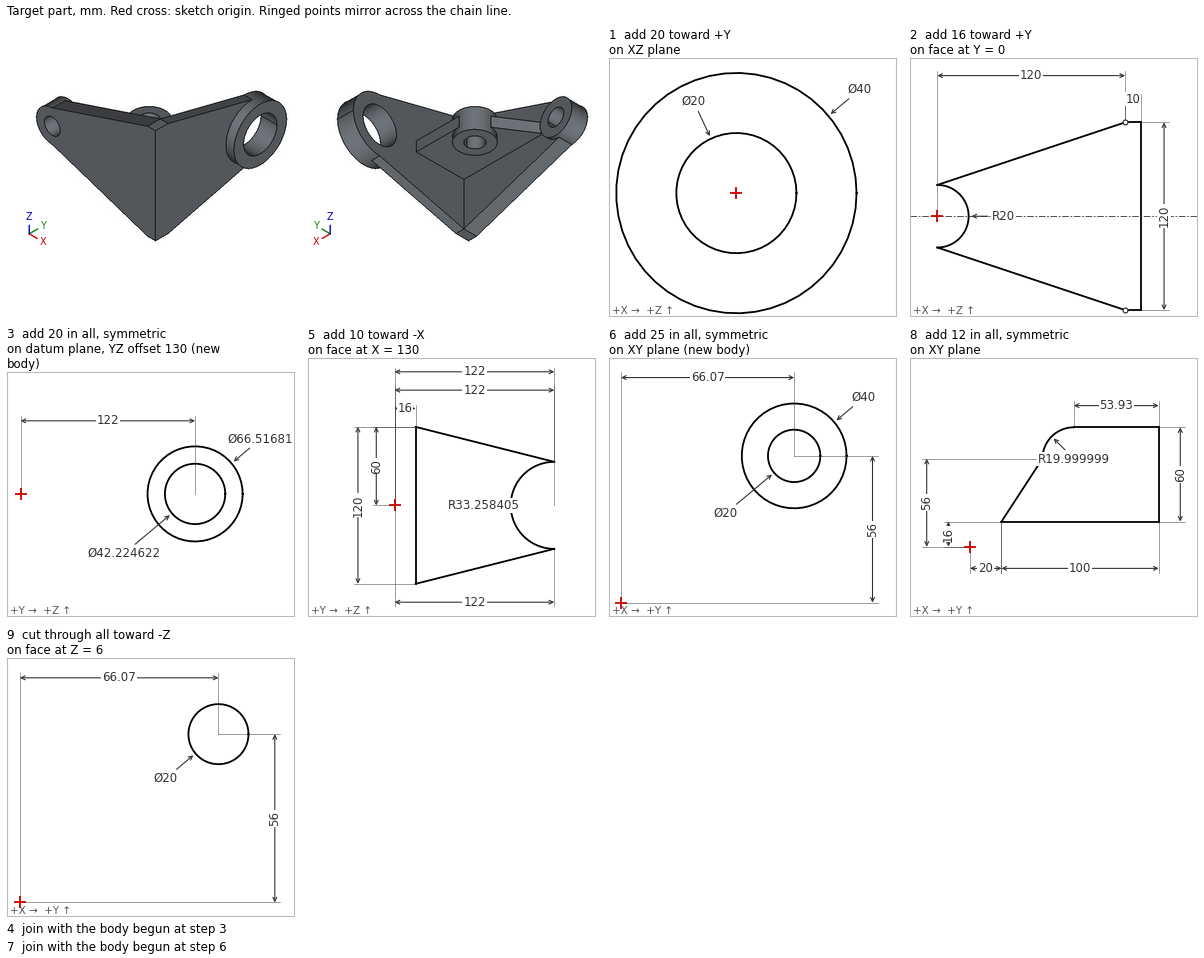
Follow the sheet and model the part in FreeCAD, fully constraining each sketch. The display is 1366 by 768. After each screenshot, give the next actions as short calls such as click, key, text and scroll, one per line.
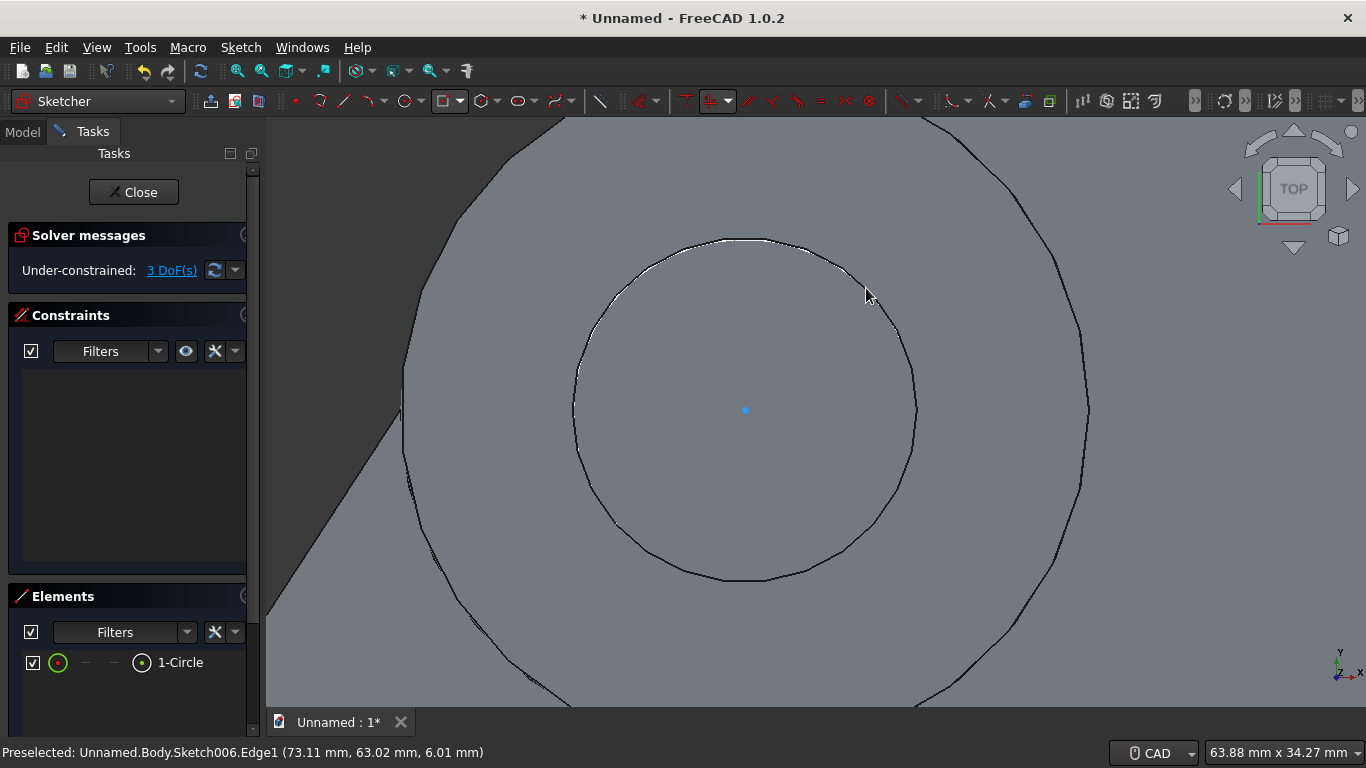
click(640, 102)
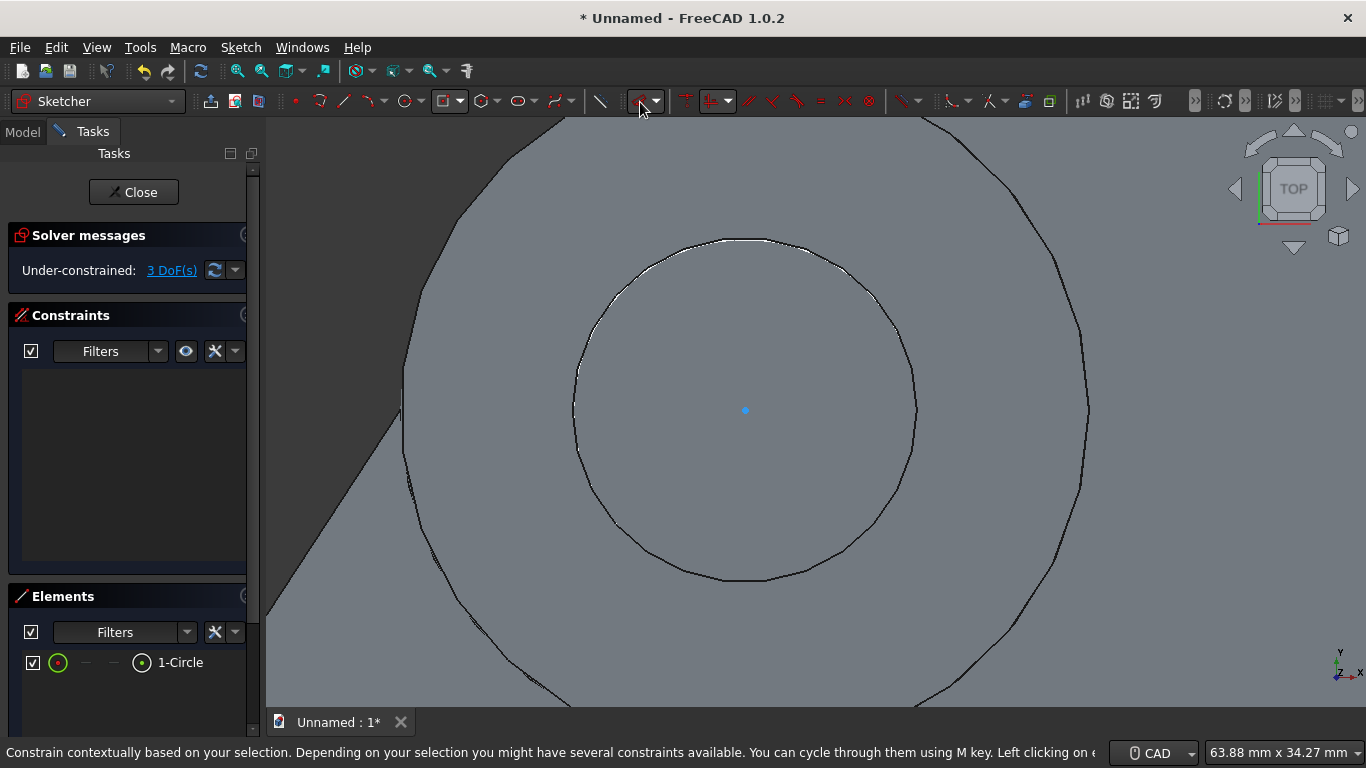
click(866, 289)
click(889, 266)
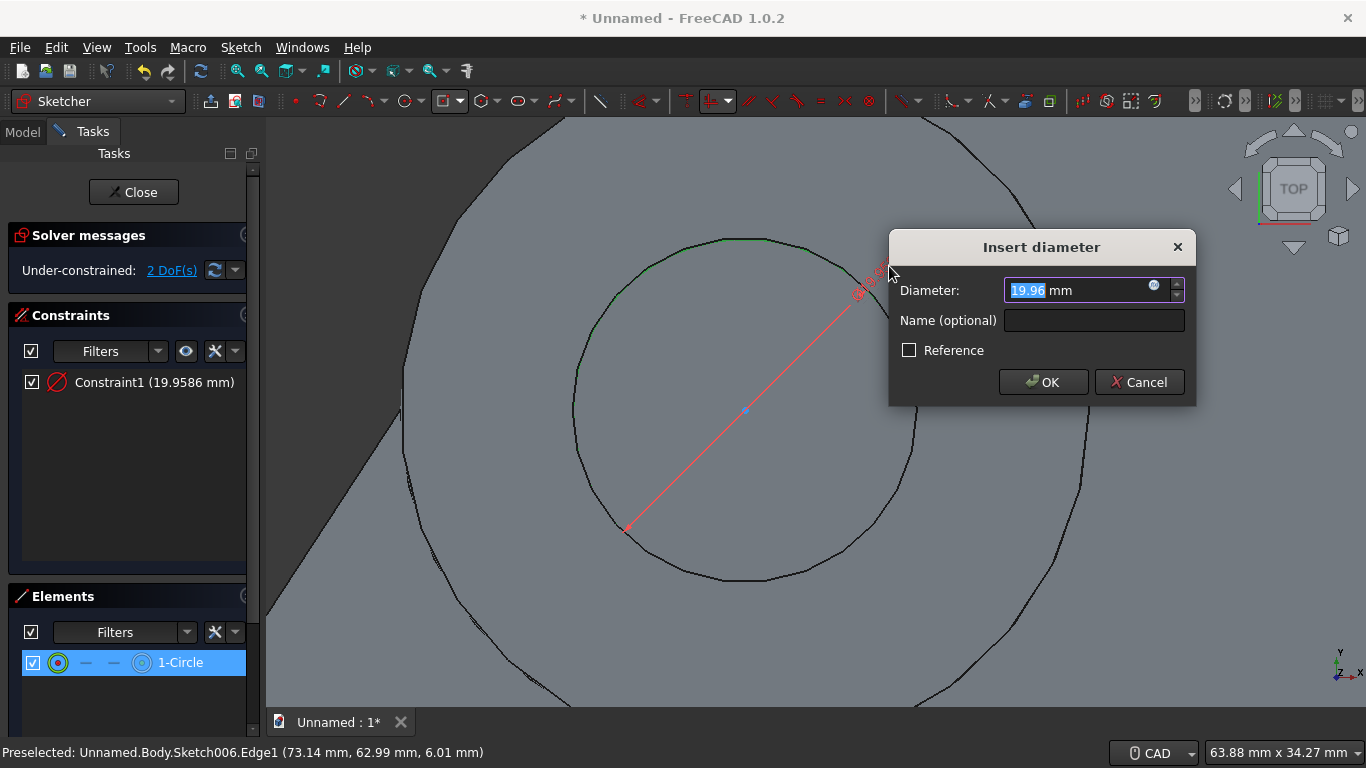
text(20)
key(Return)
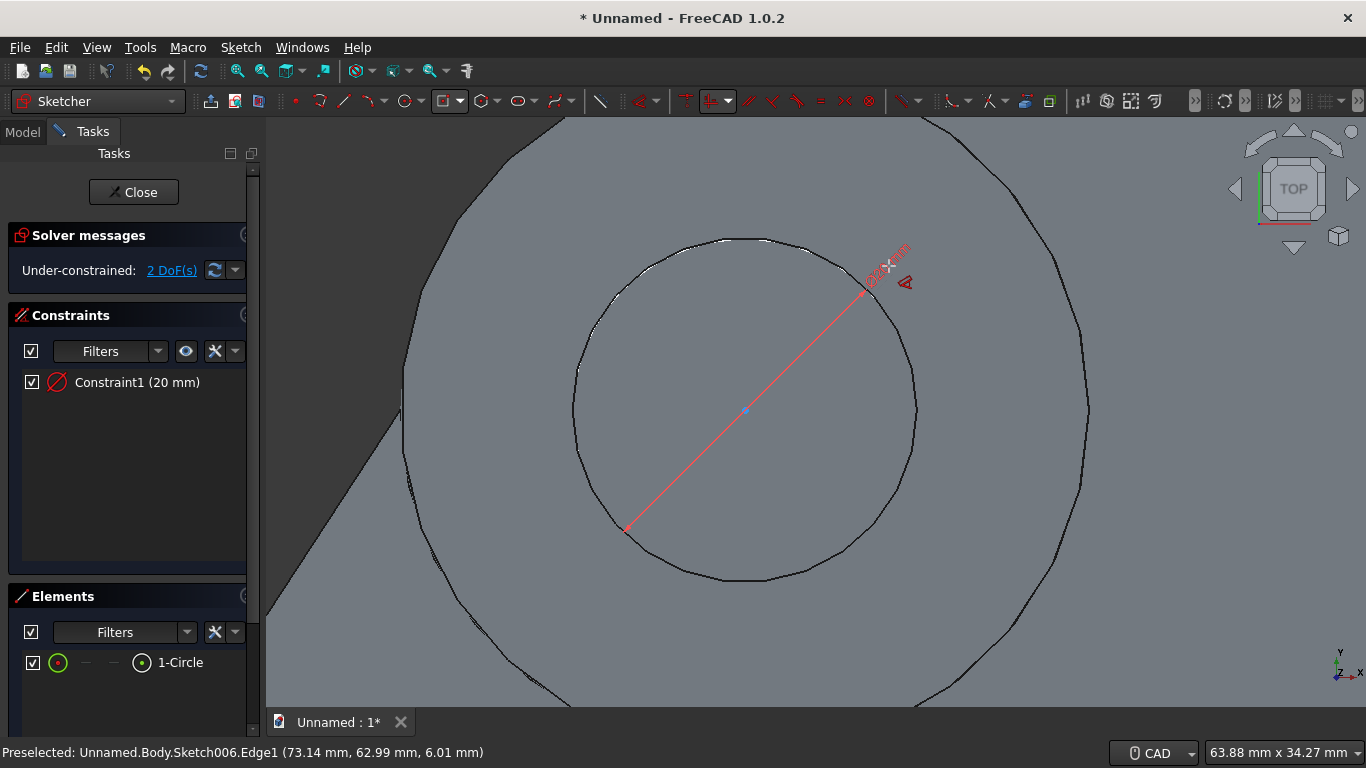
click(745, 411)
click(779, 545)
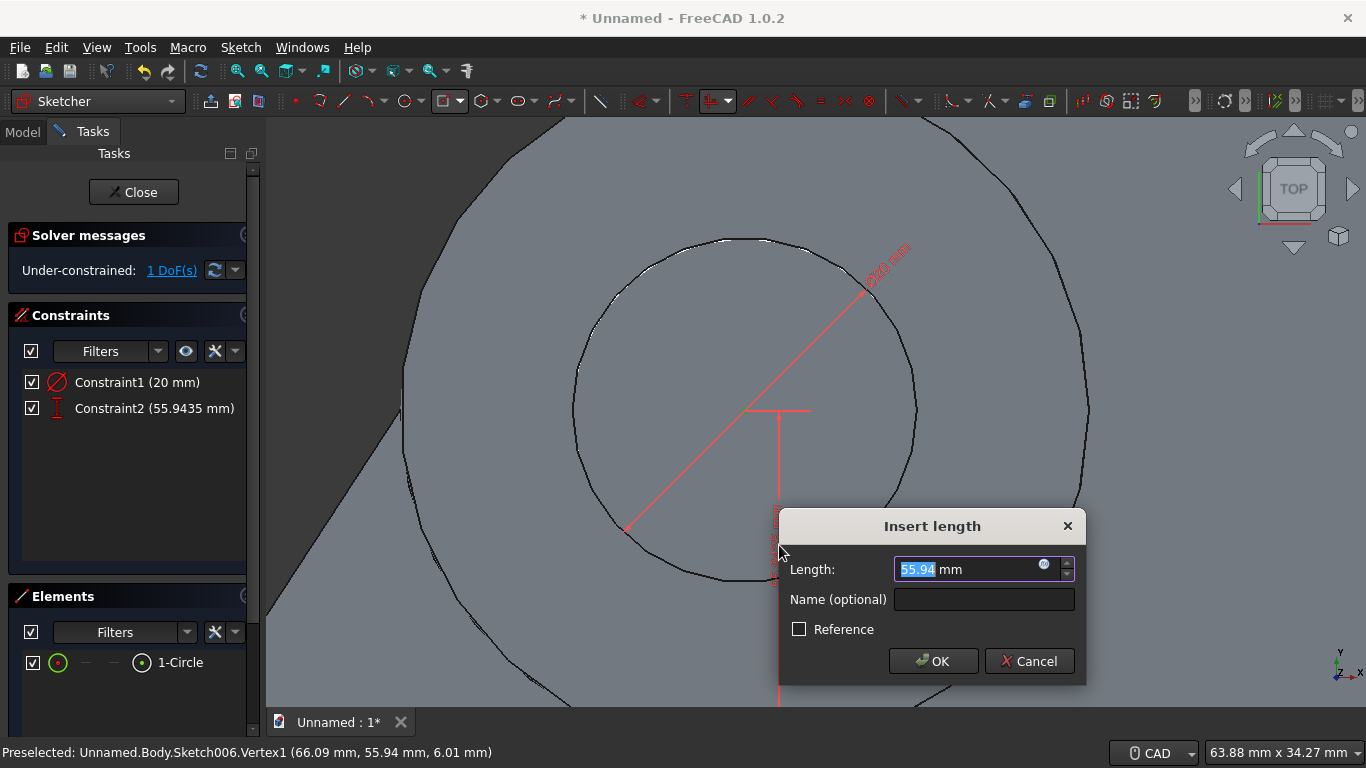
text(56)
key(Return)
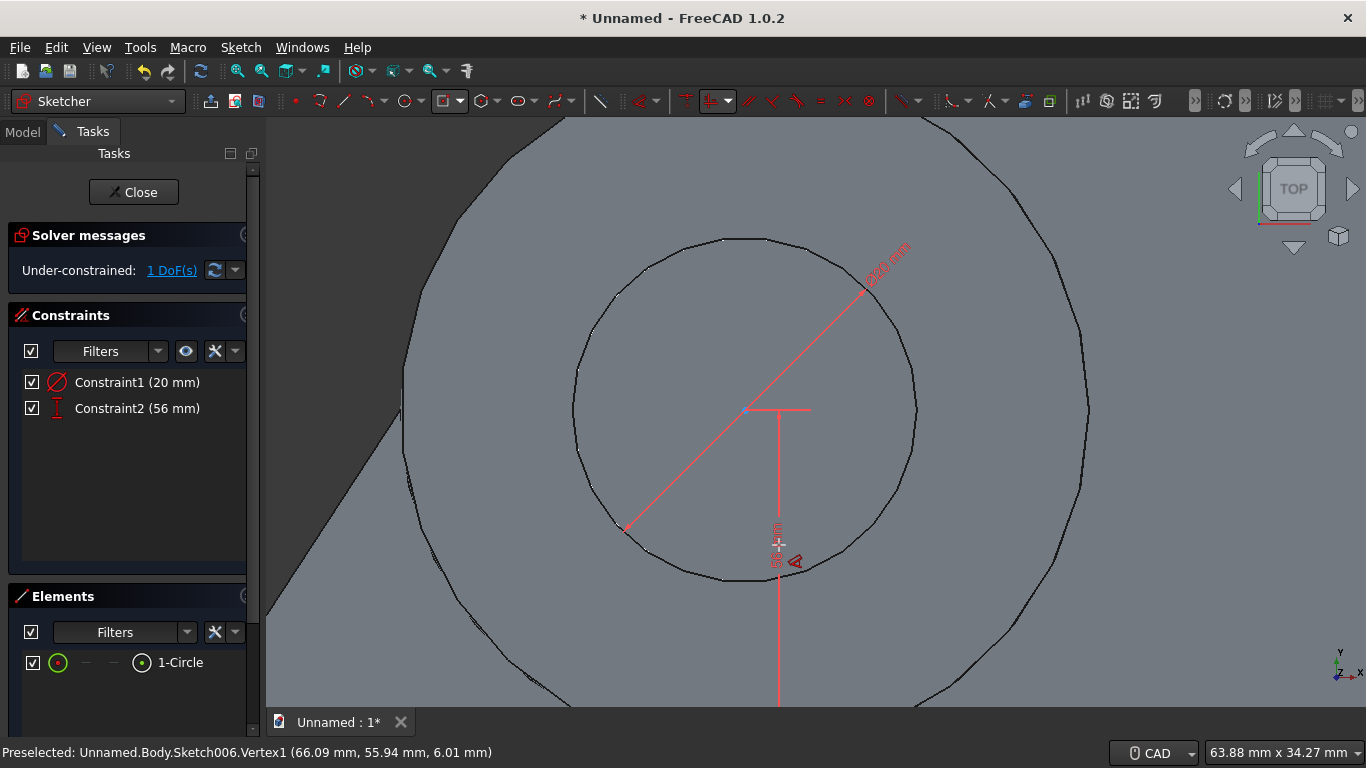
click(745, 410)
click(519, 376)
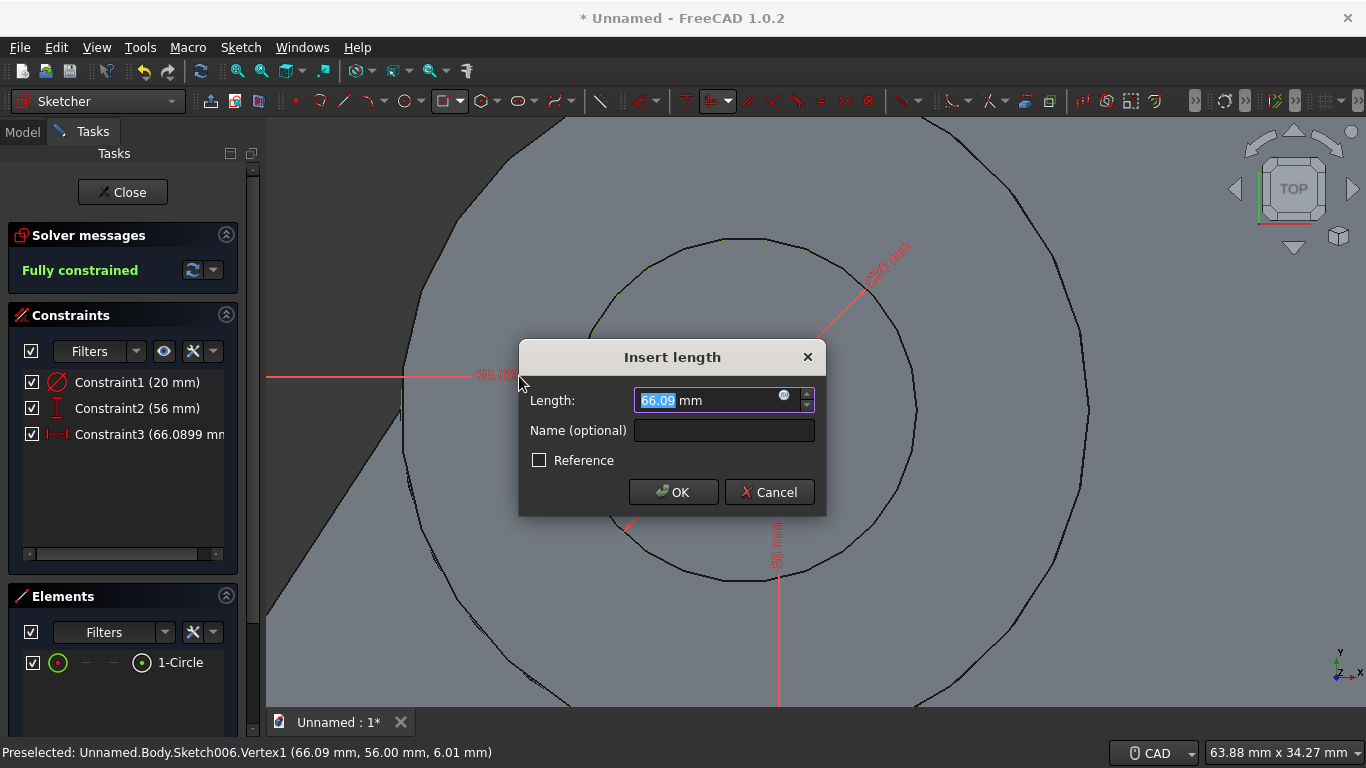
text(66.07)
key(Return)
key(Escape)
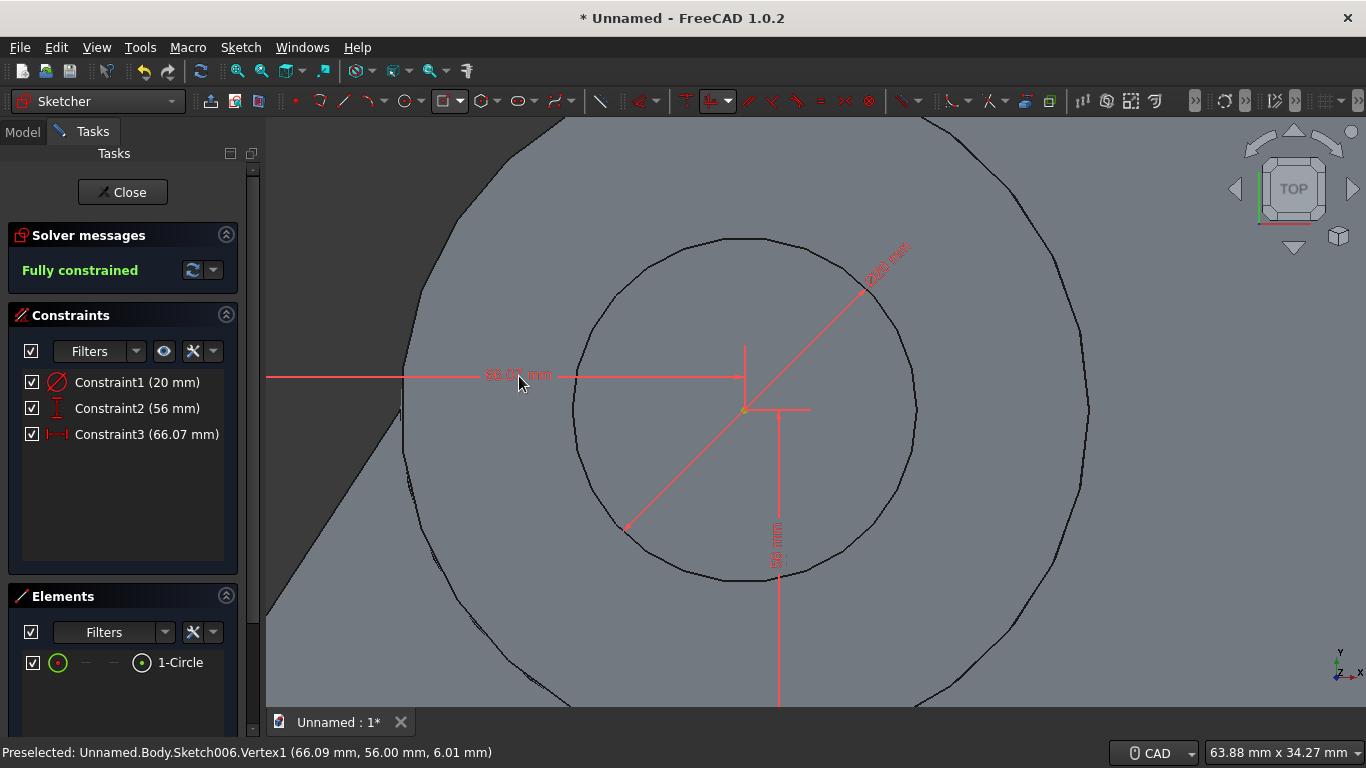
click(123, 192)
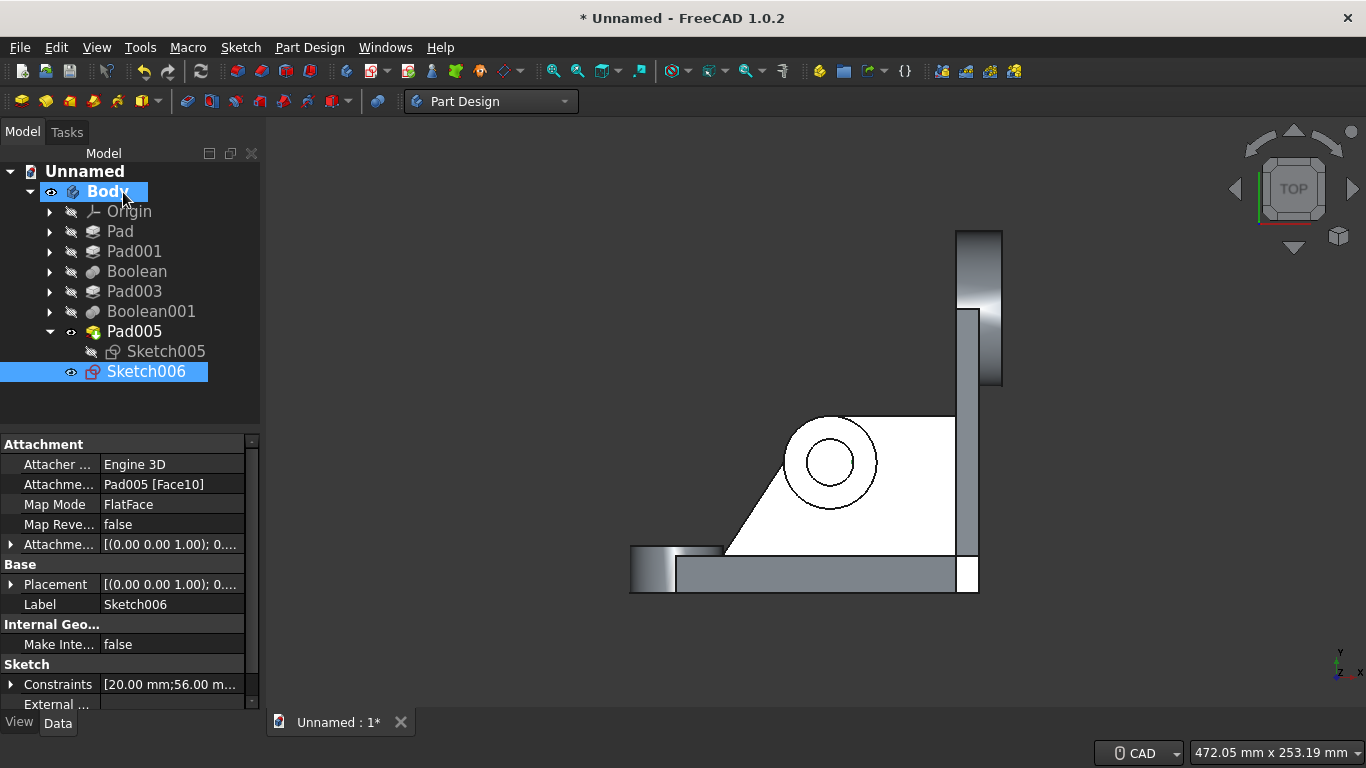
click(188, 102)